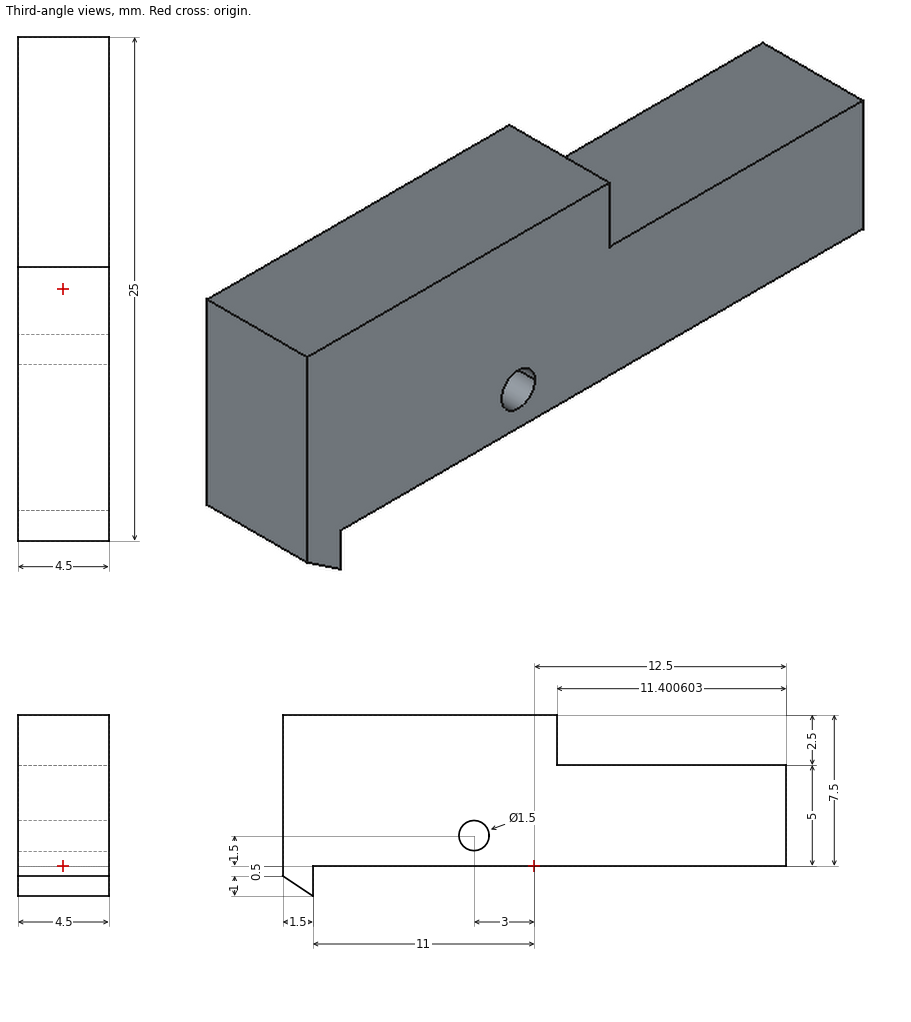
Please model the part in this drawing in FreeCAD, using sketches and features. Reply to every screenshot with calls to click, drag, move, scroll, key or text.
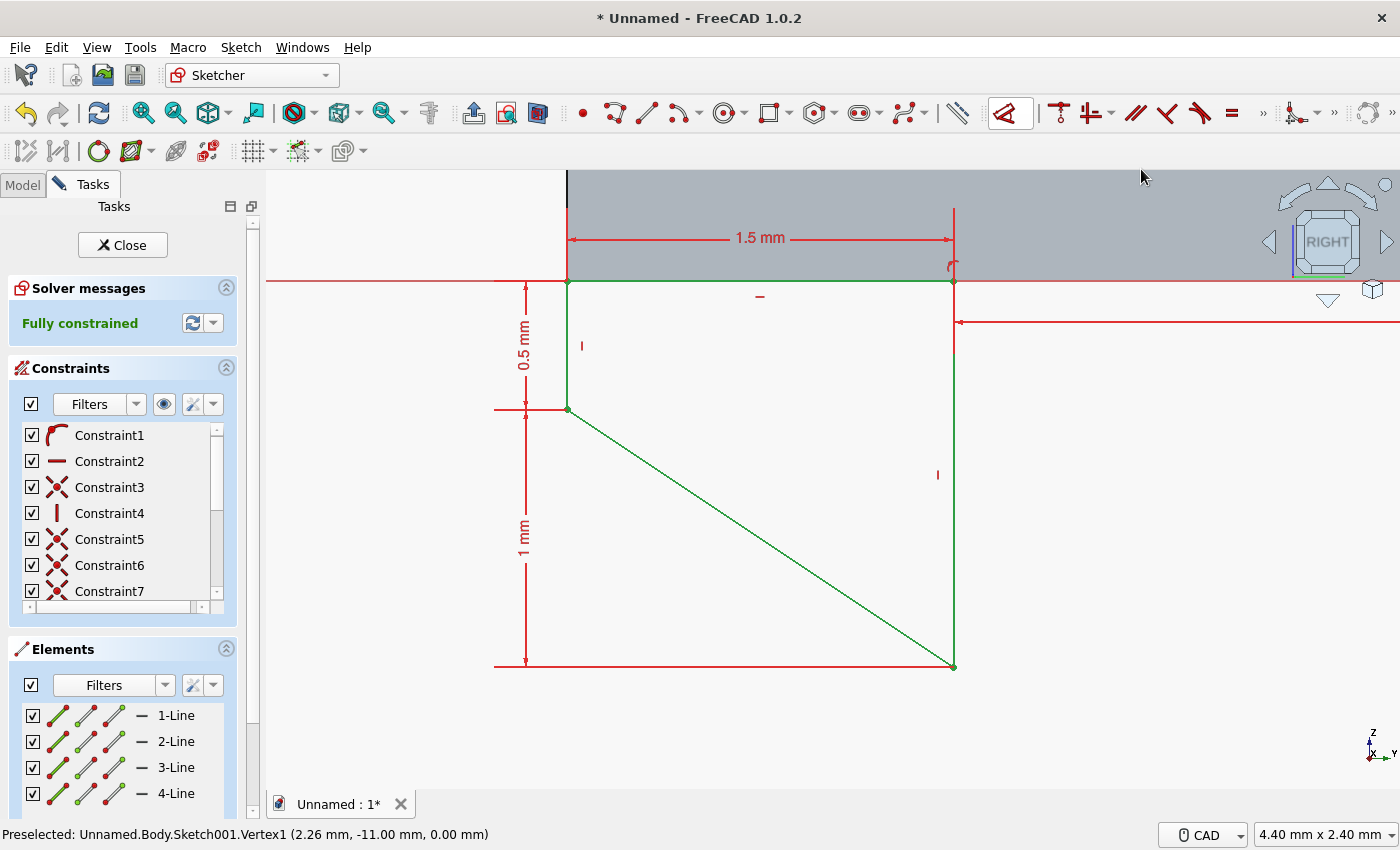
click(123, 245)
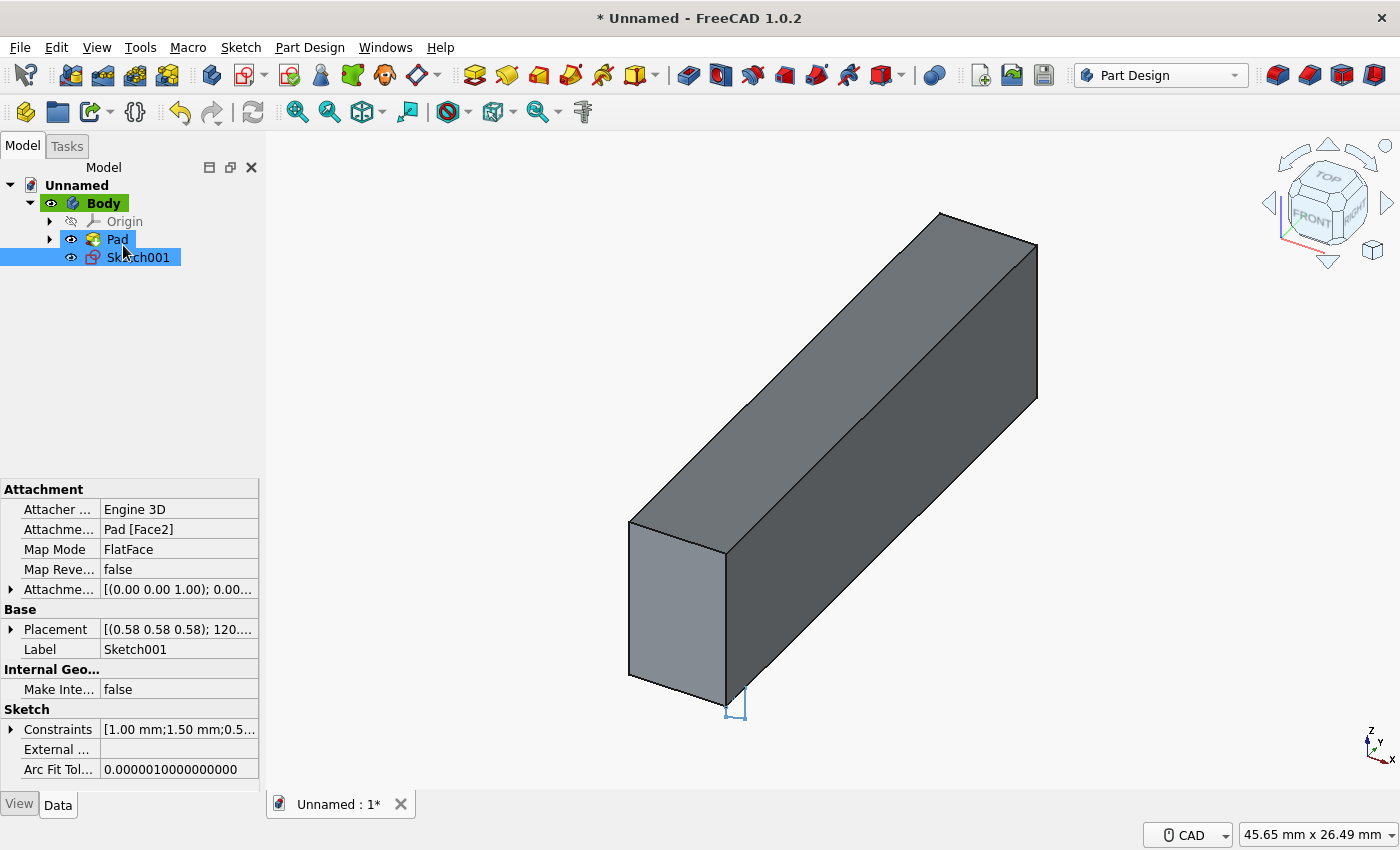
click(476, 76)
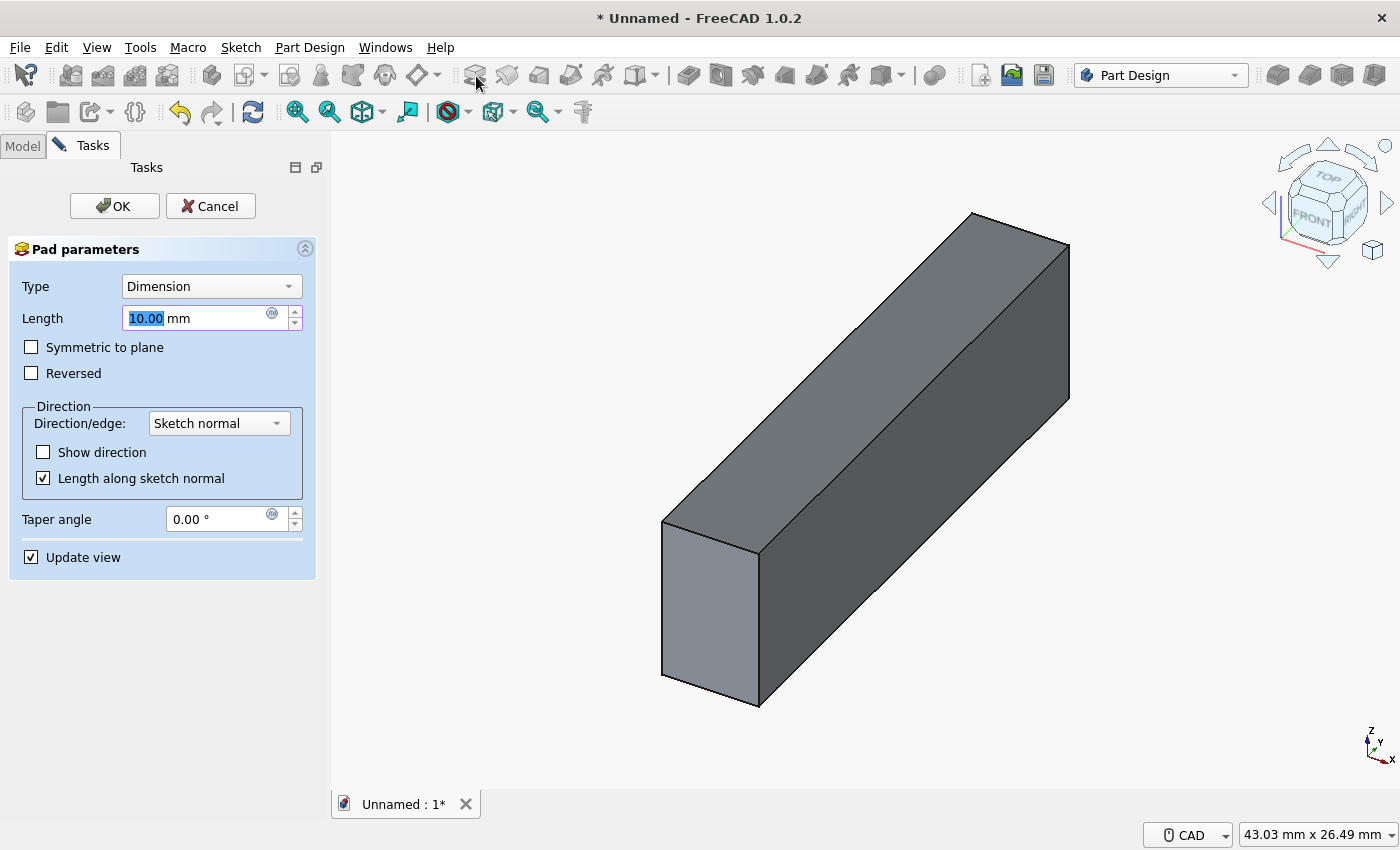
text(4.5)
key(Tab)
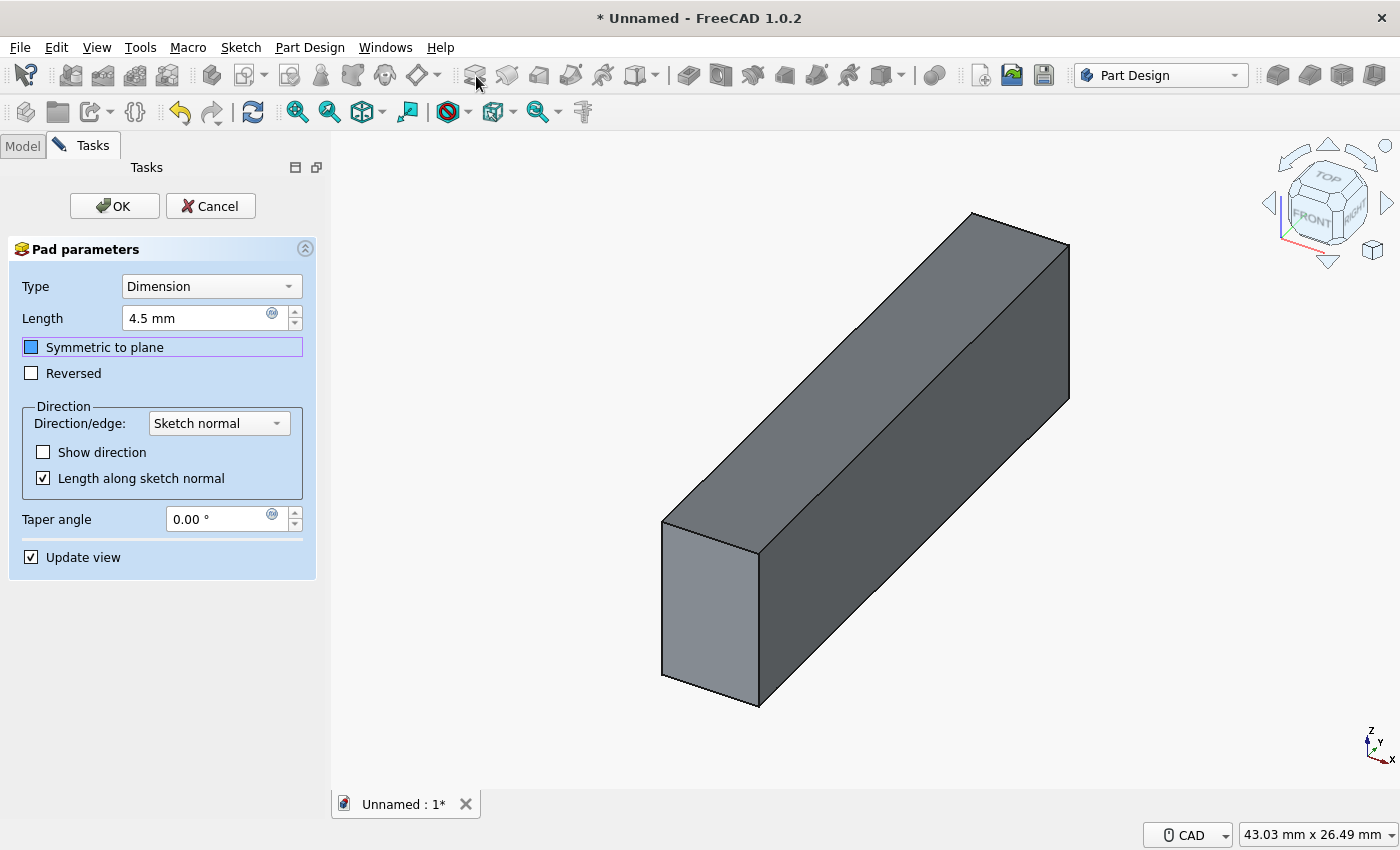
click(30, 373)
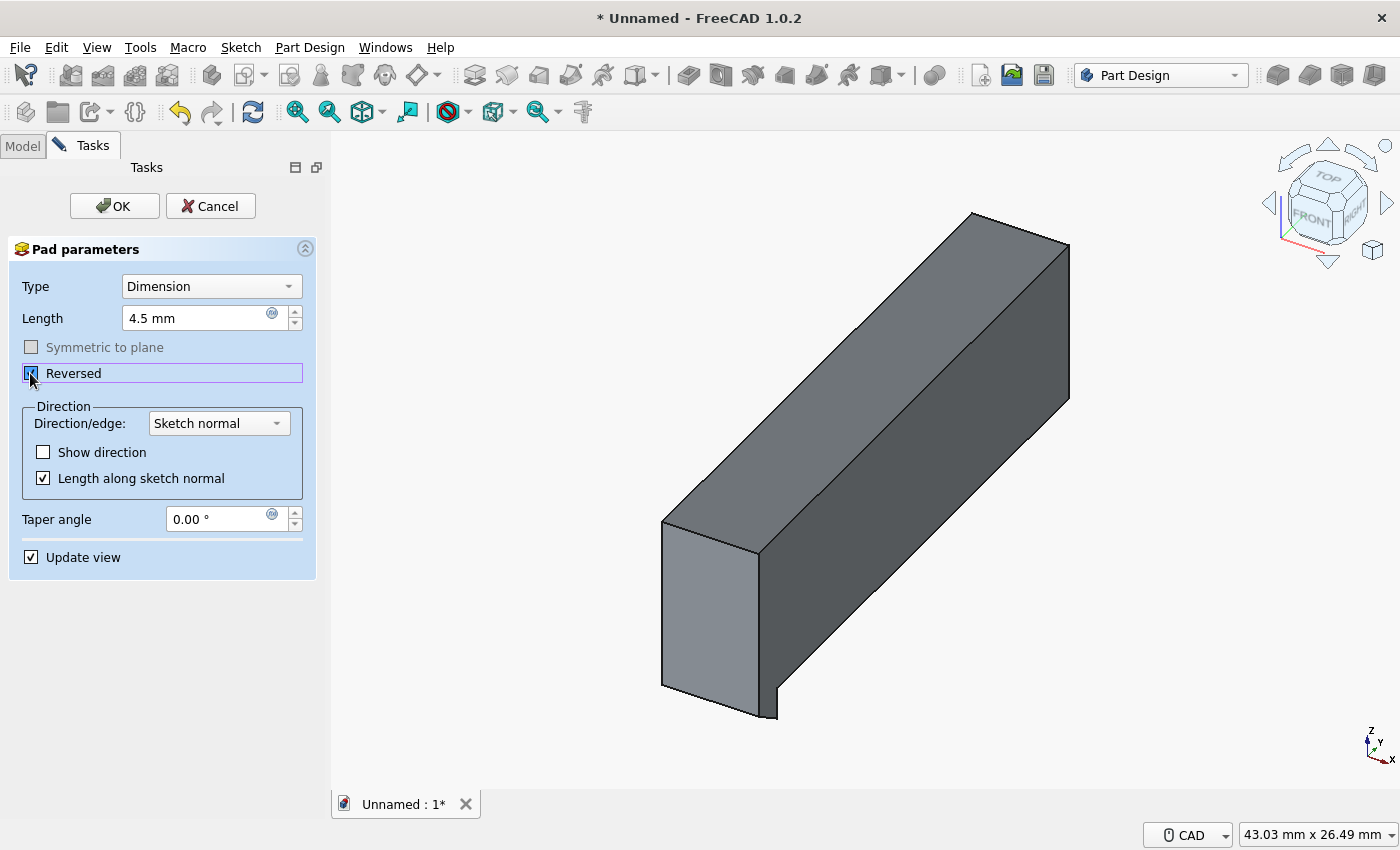
click(115, 206)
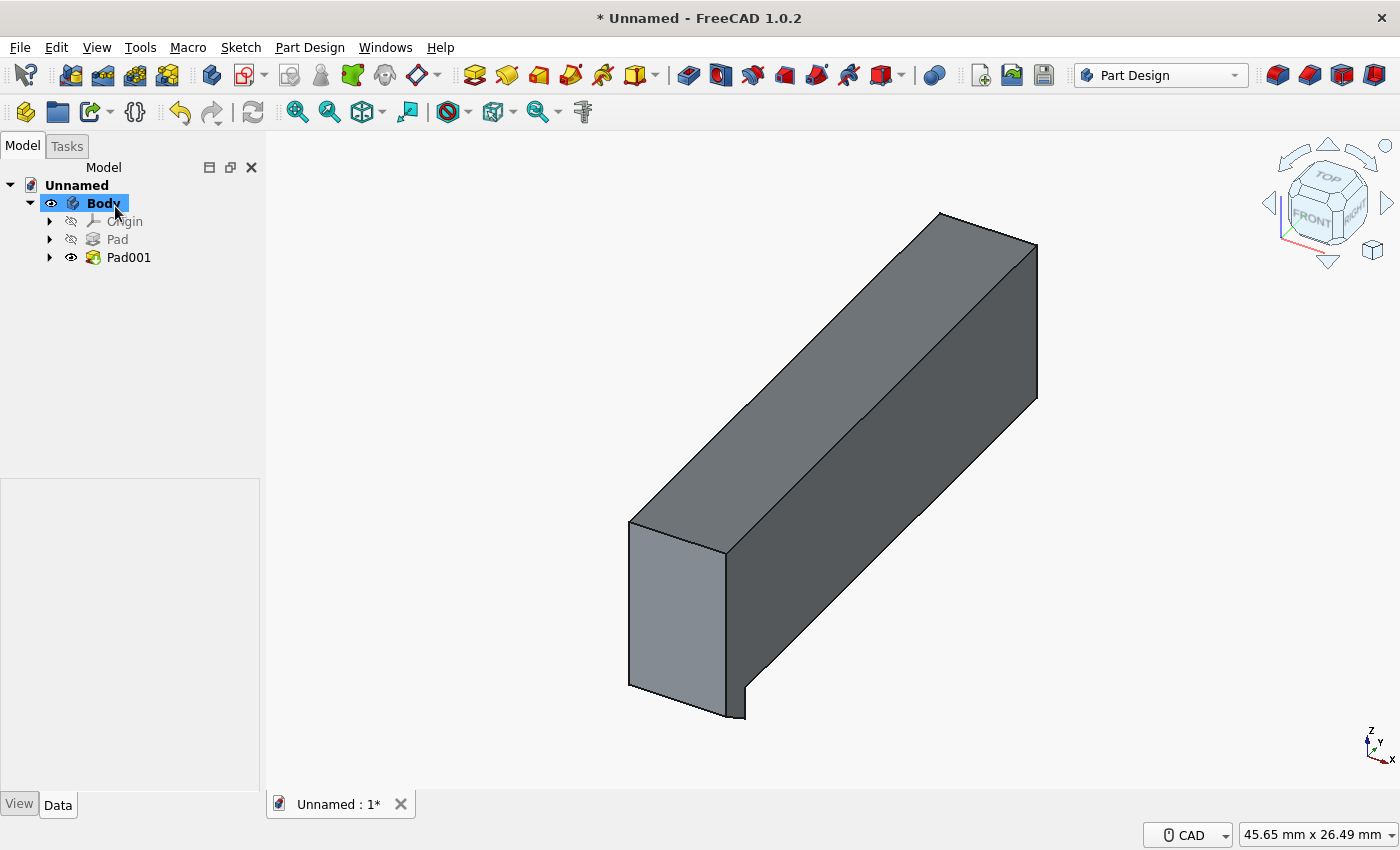
click(970, 376)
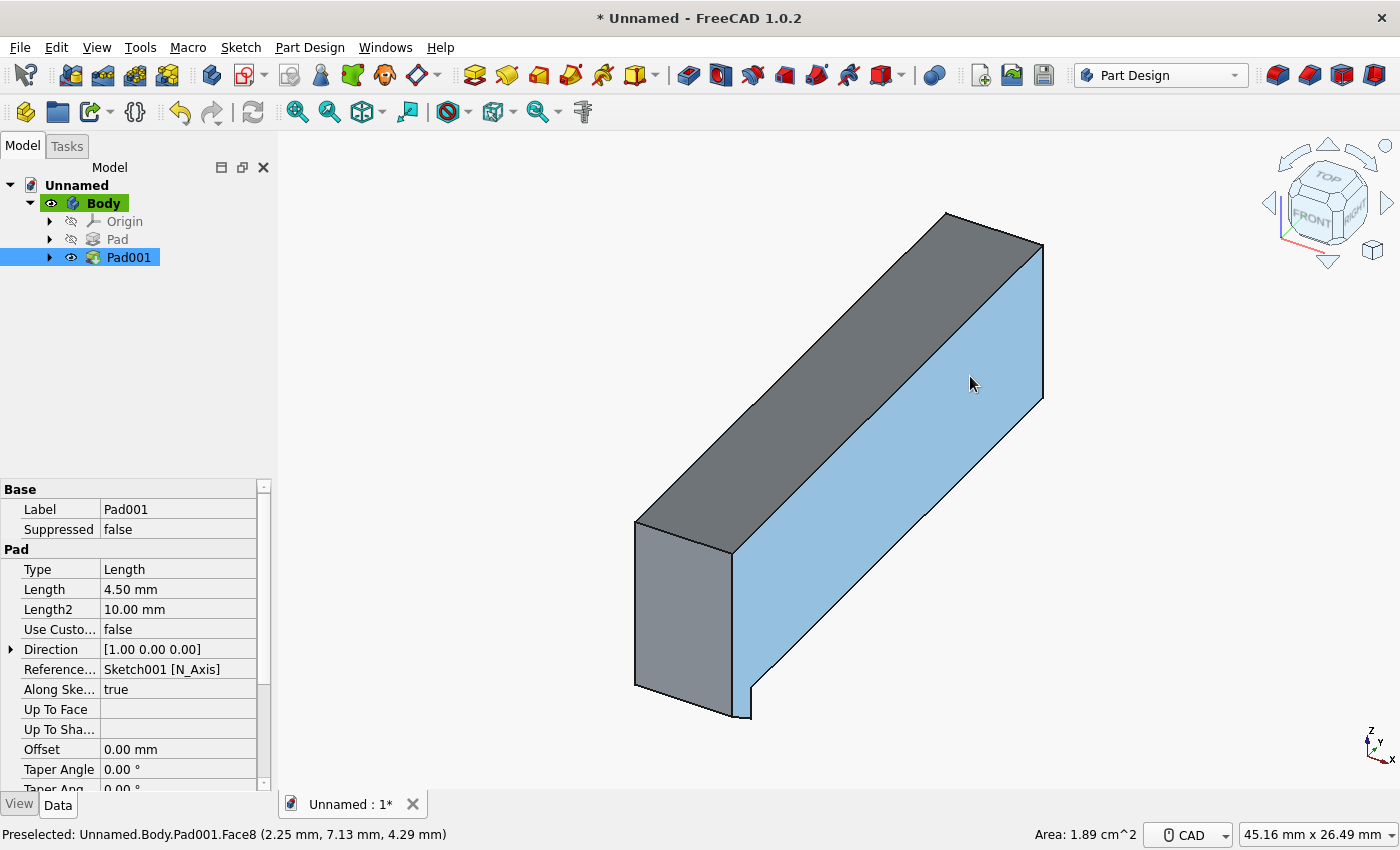
click(244, 76)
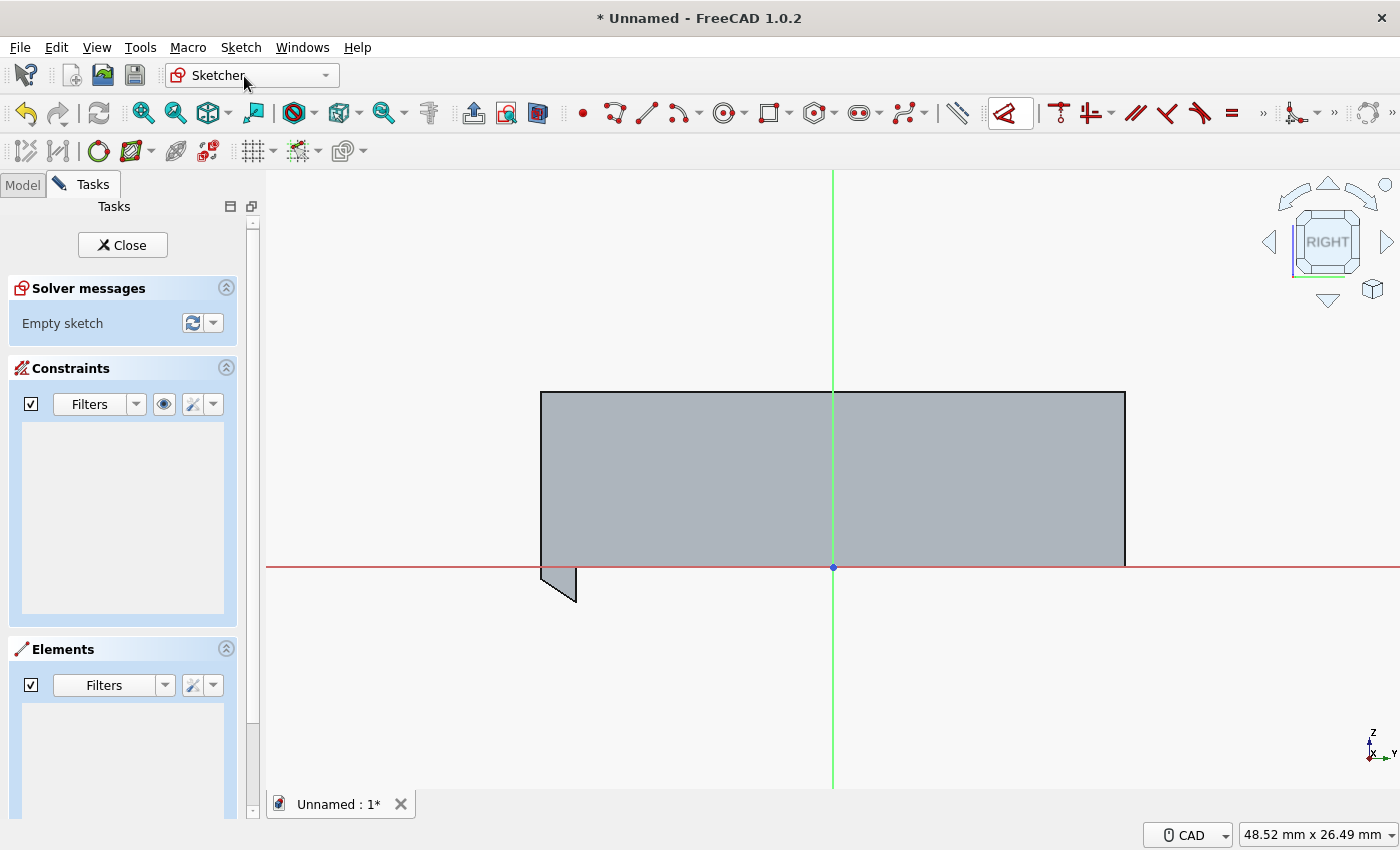
scroll(763, 537, up, 12)